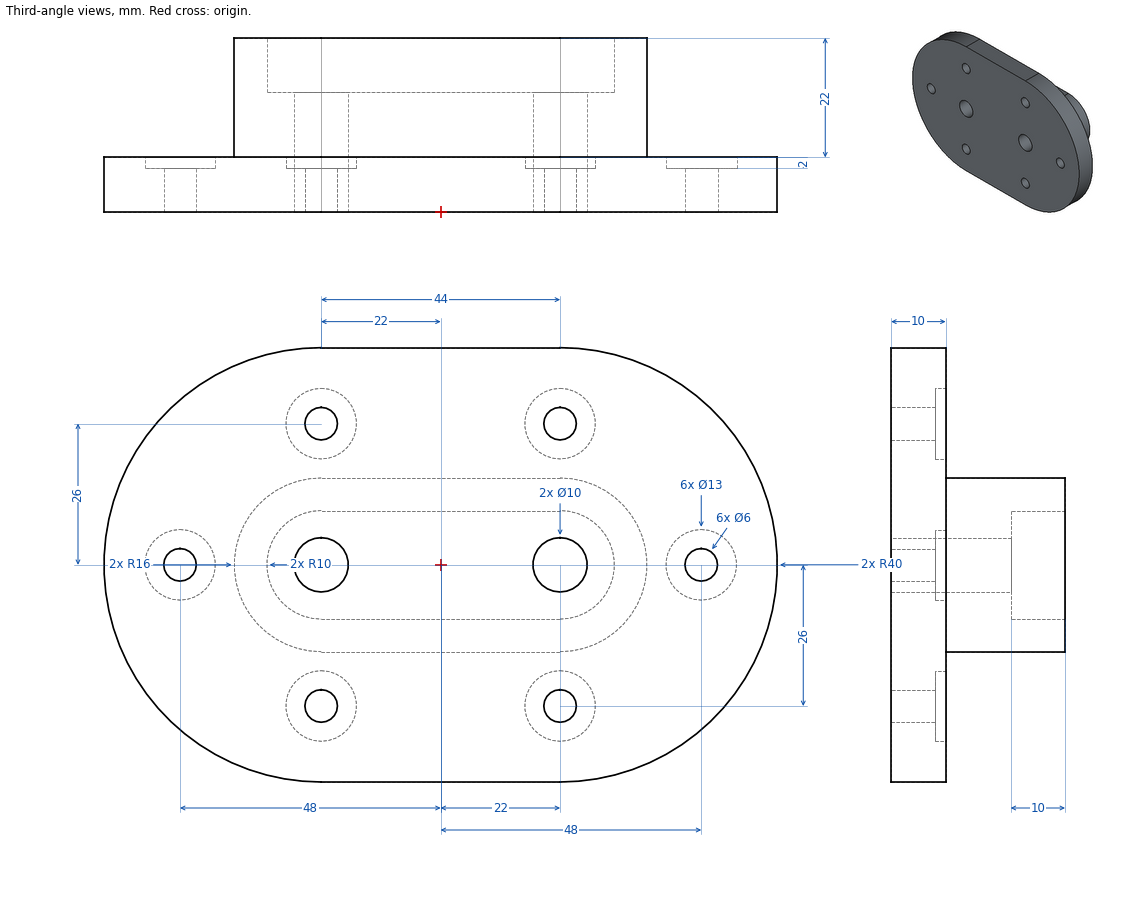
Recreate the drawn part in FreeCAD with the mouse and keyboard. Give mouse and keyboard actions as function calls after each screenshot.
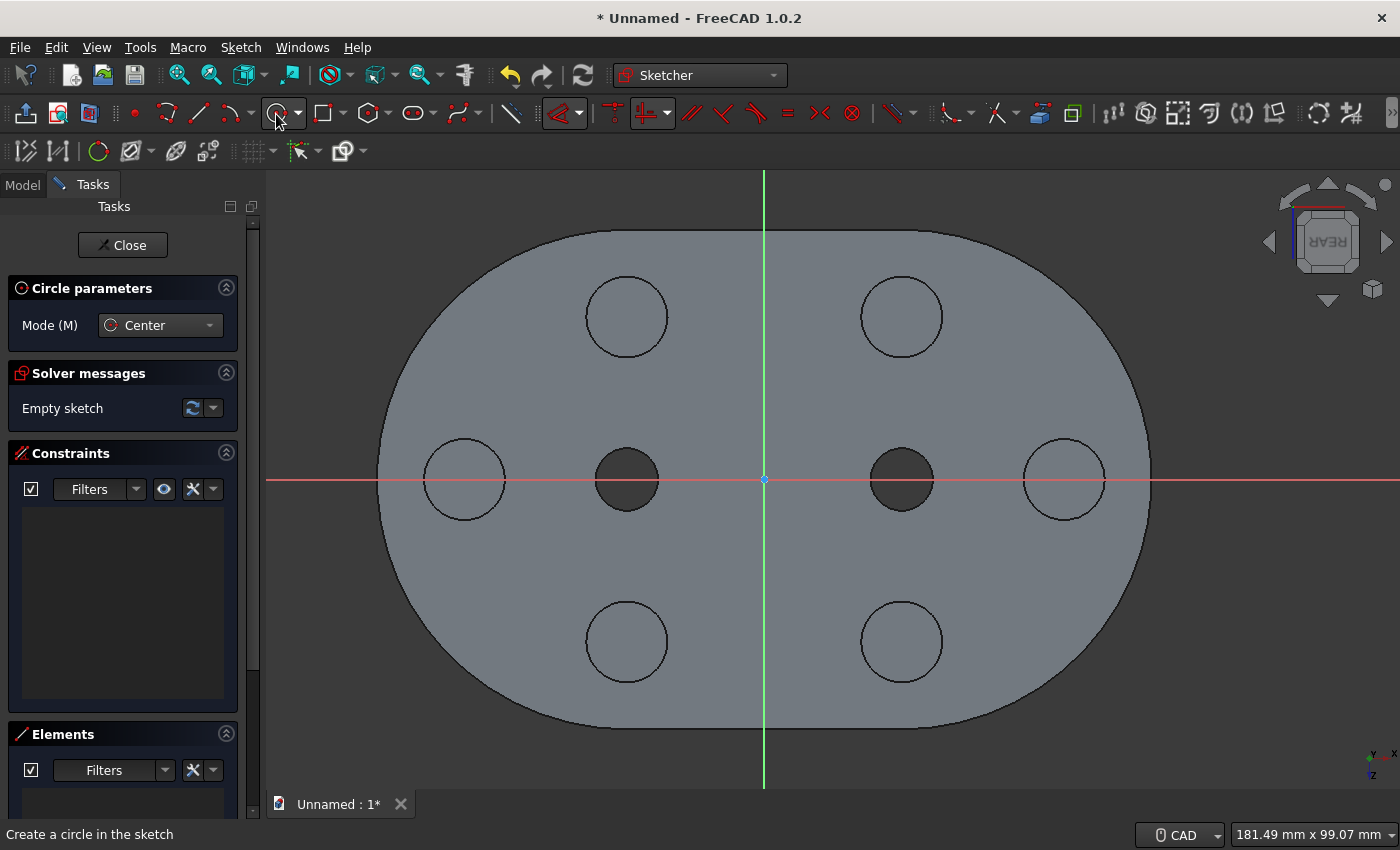
click(1064, 479)
click(1071, 462)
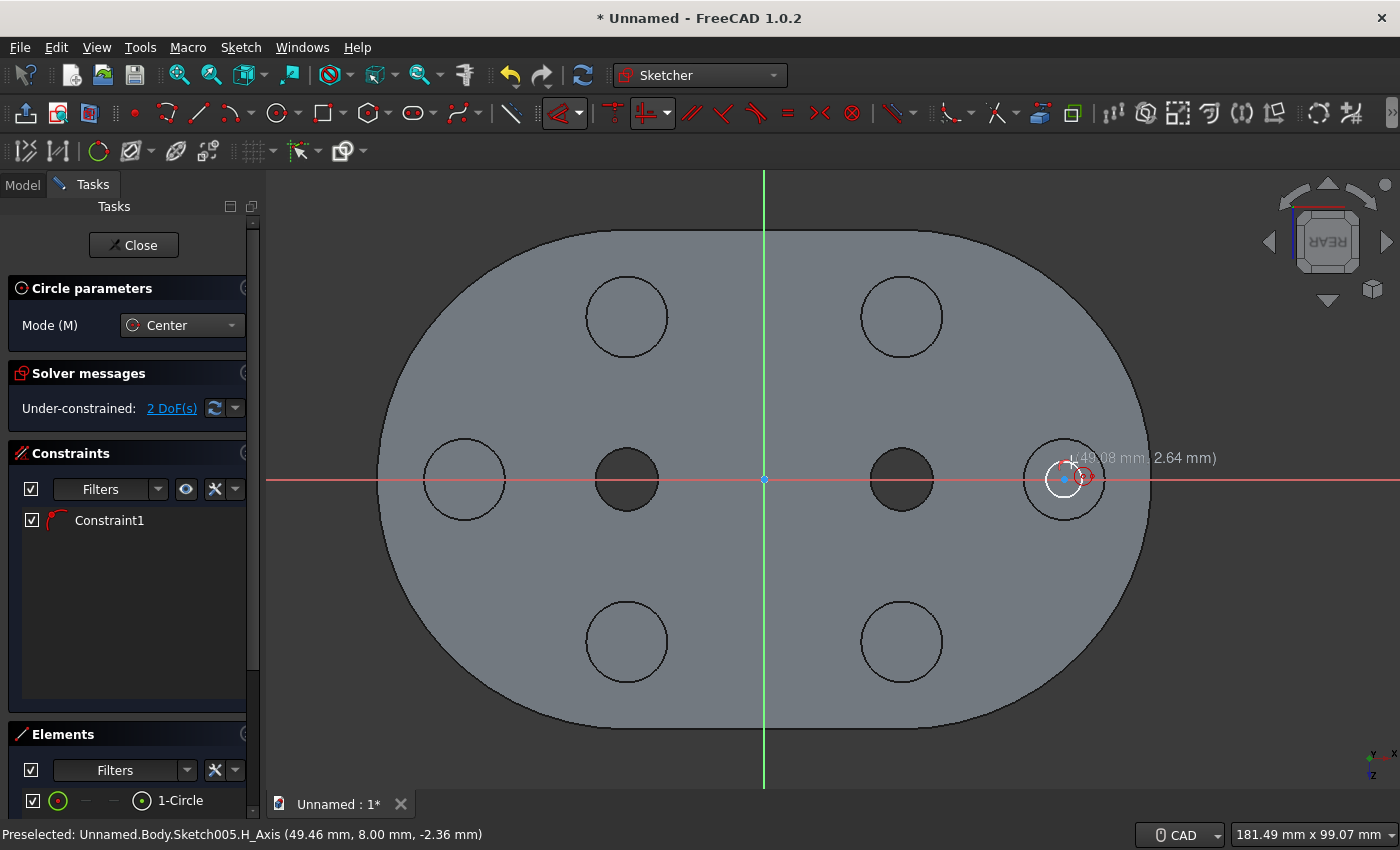
click(902, 642)
click(915, 629)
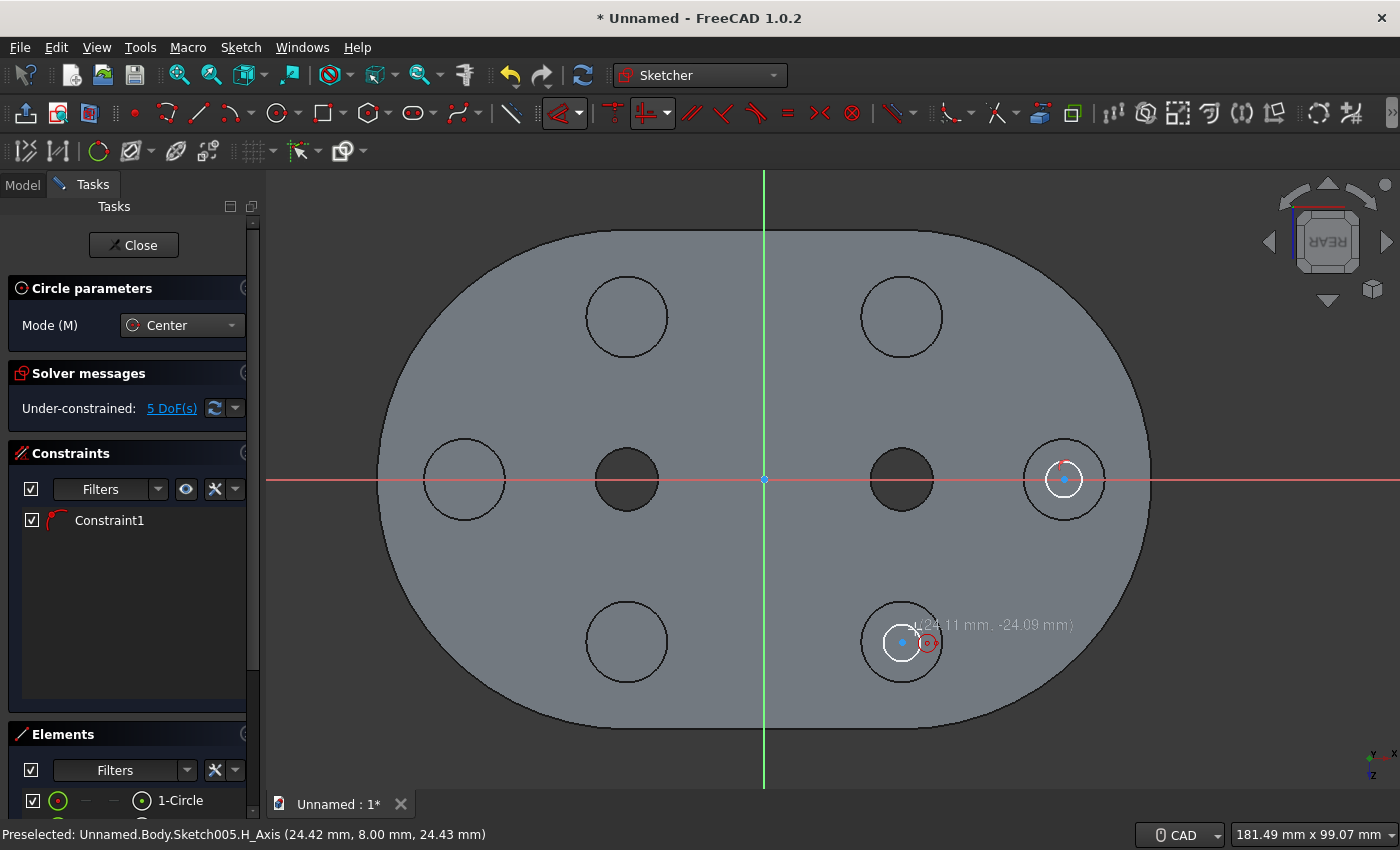
click(627, 642)
click(640, 629)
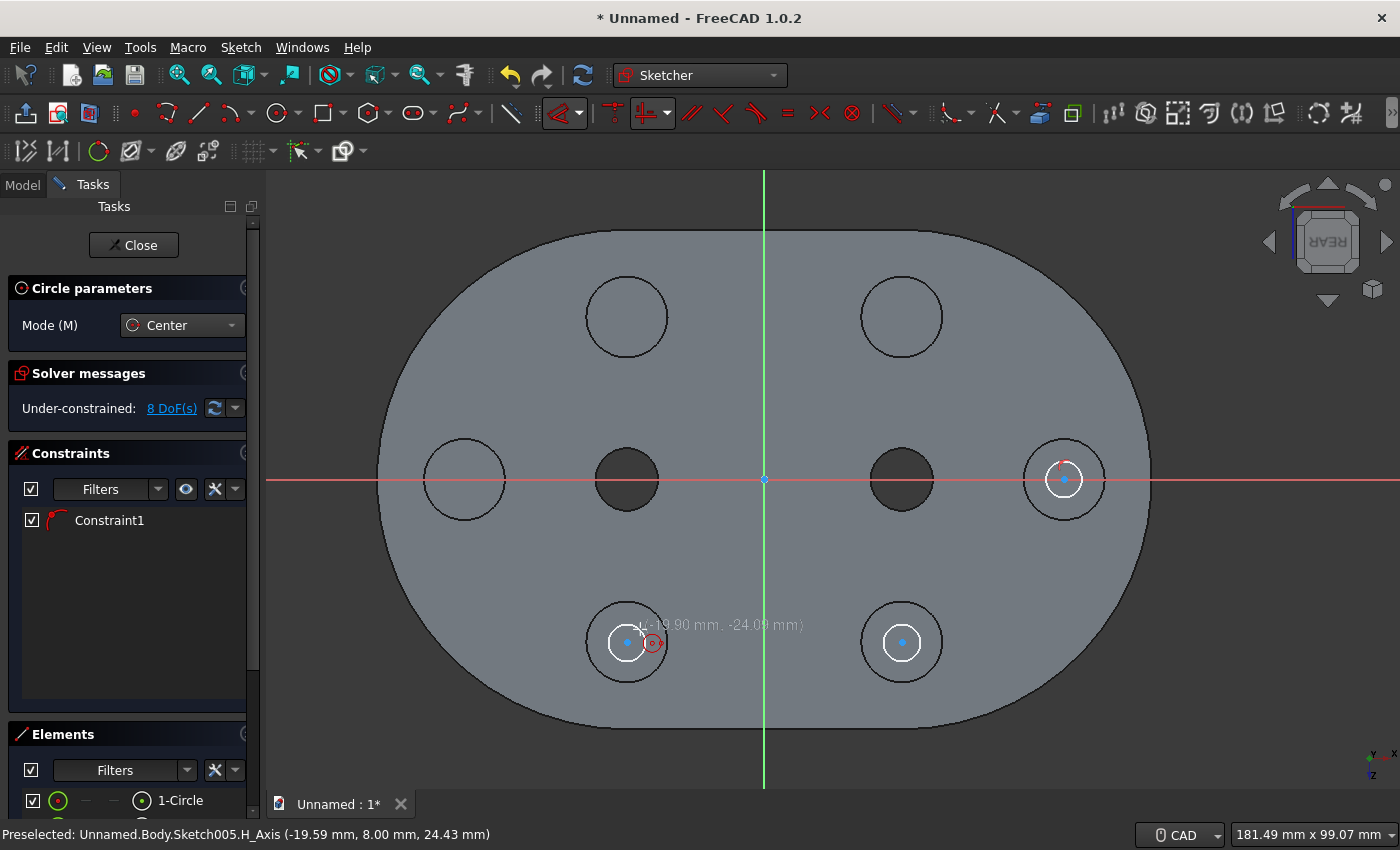
click(464, 479)
click(471, 462)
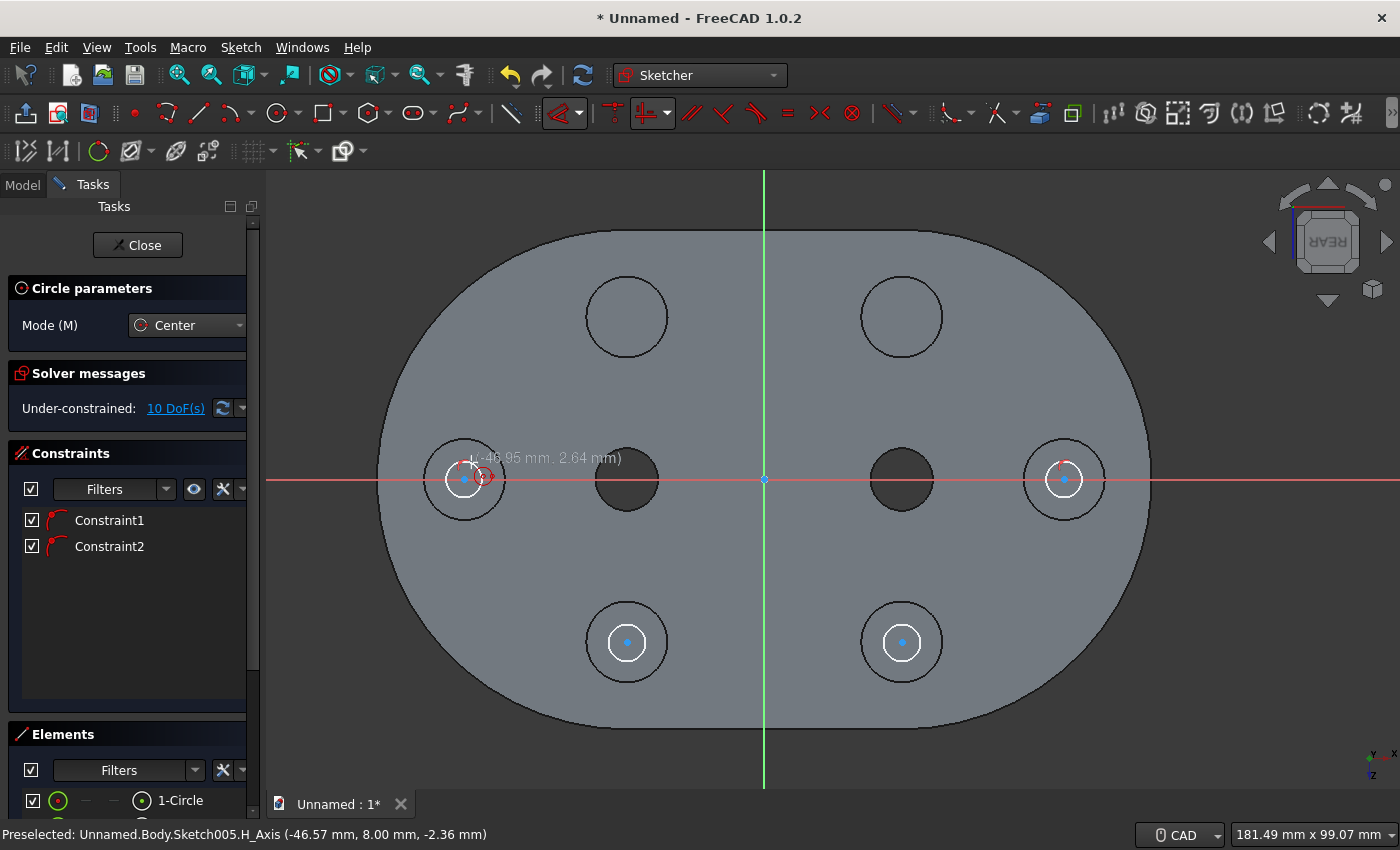
click(627, 317)
click(640, 304)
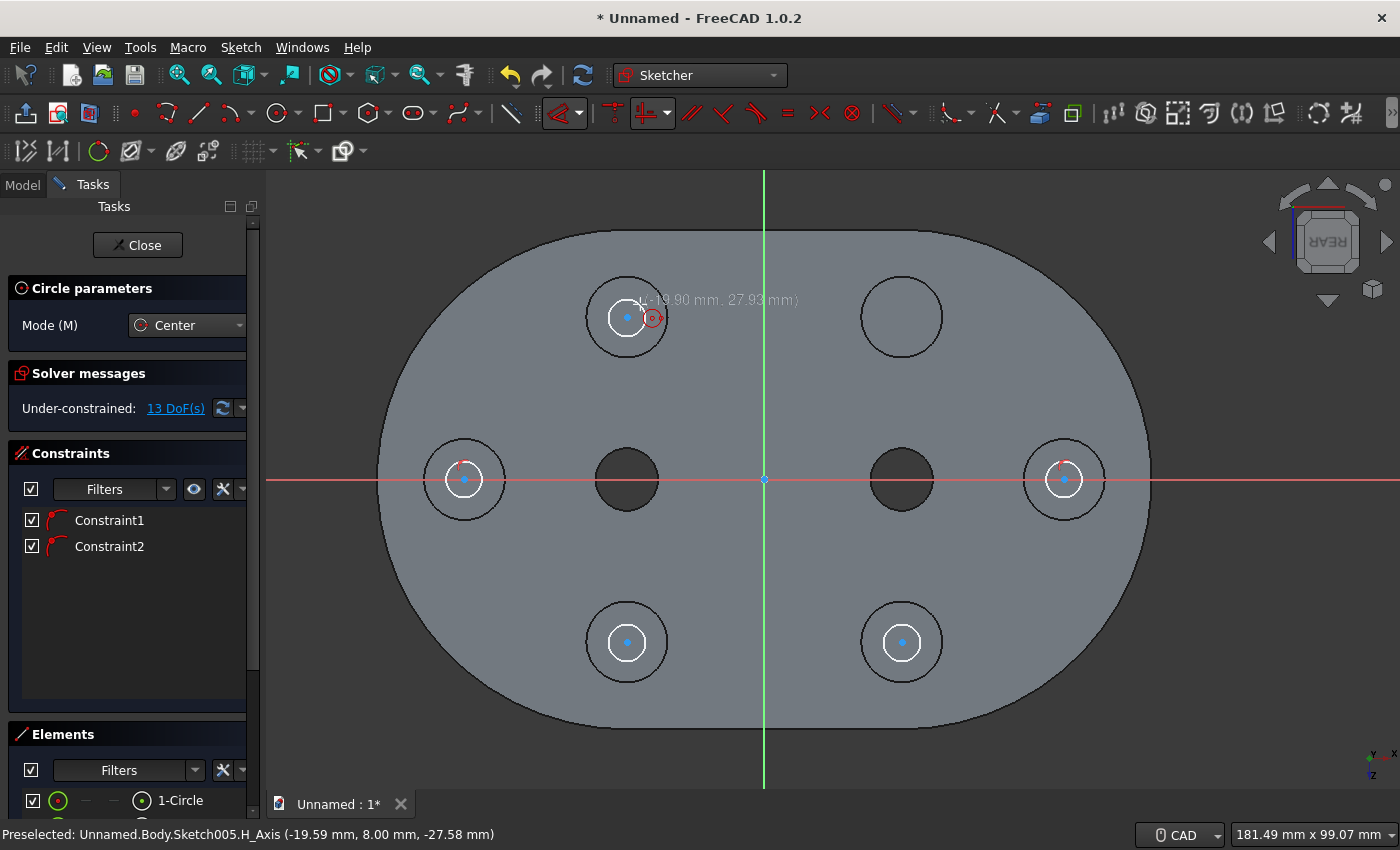
click(902, 317)
click(915, 304)
key(Escape)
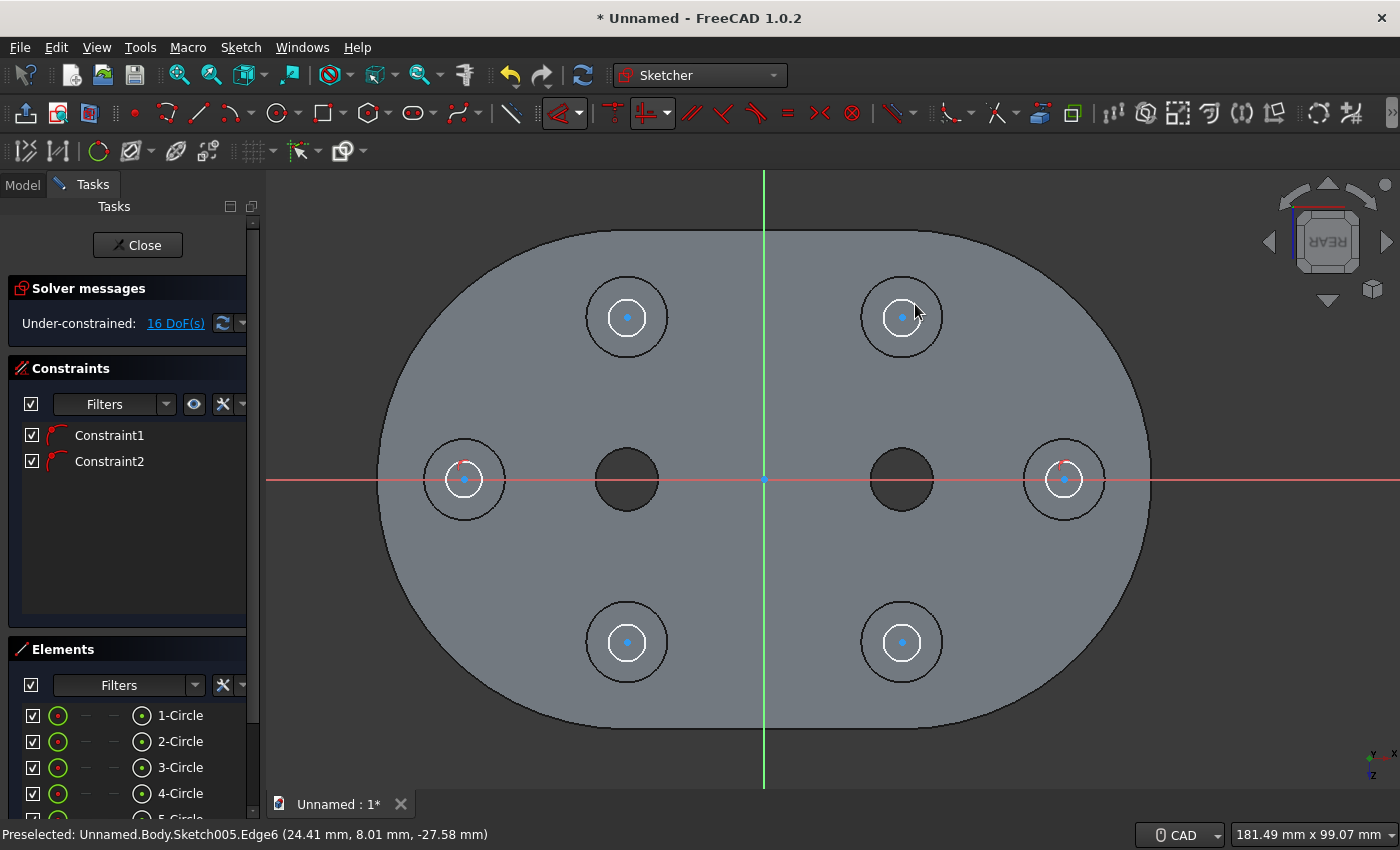
click(1077, 467)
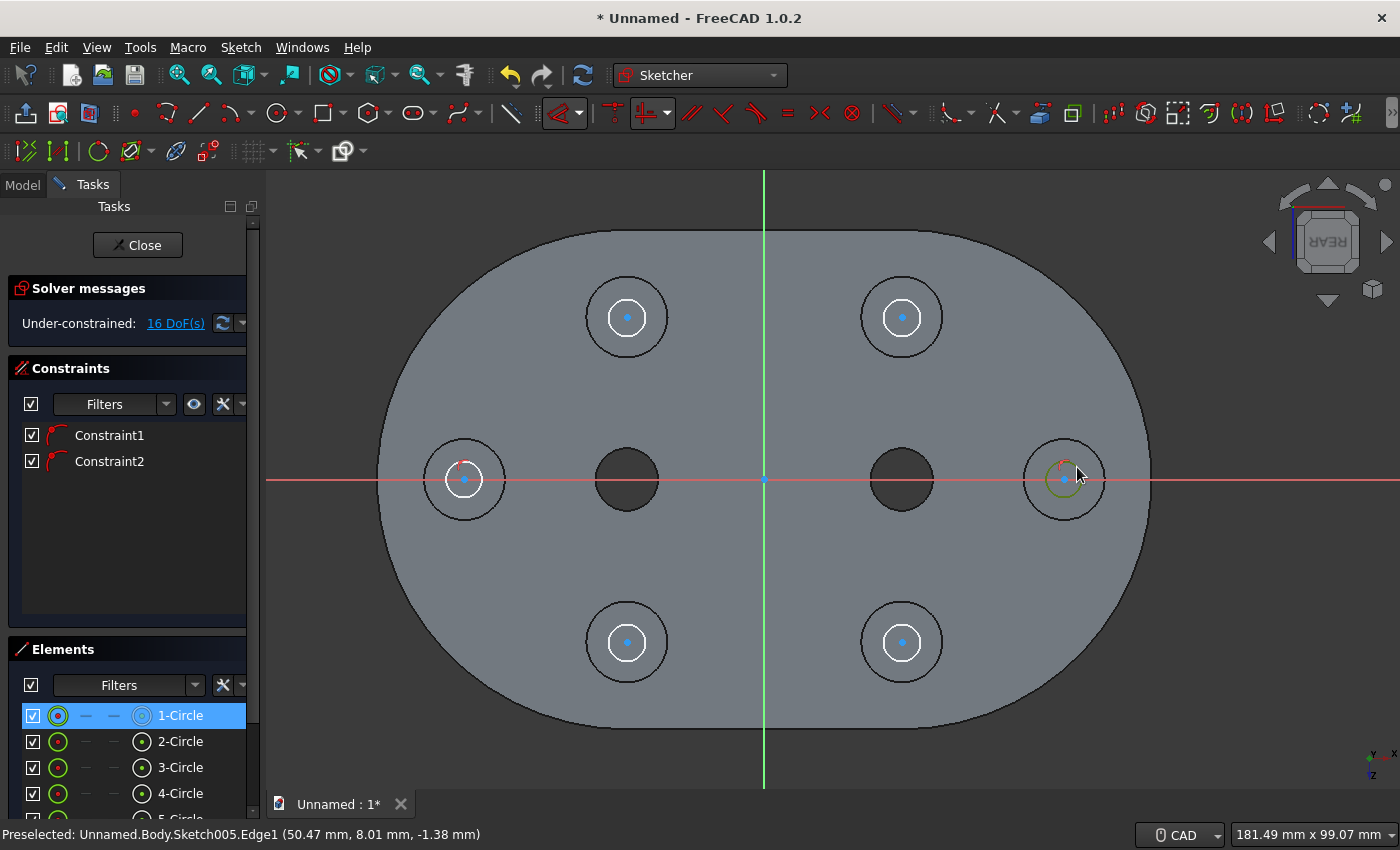
click(915, 630)